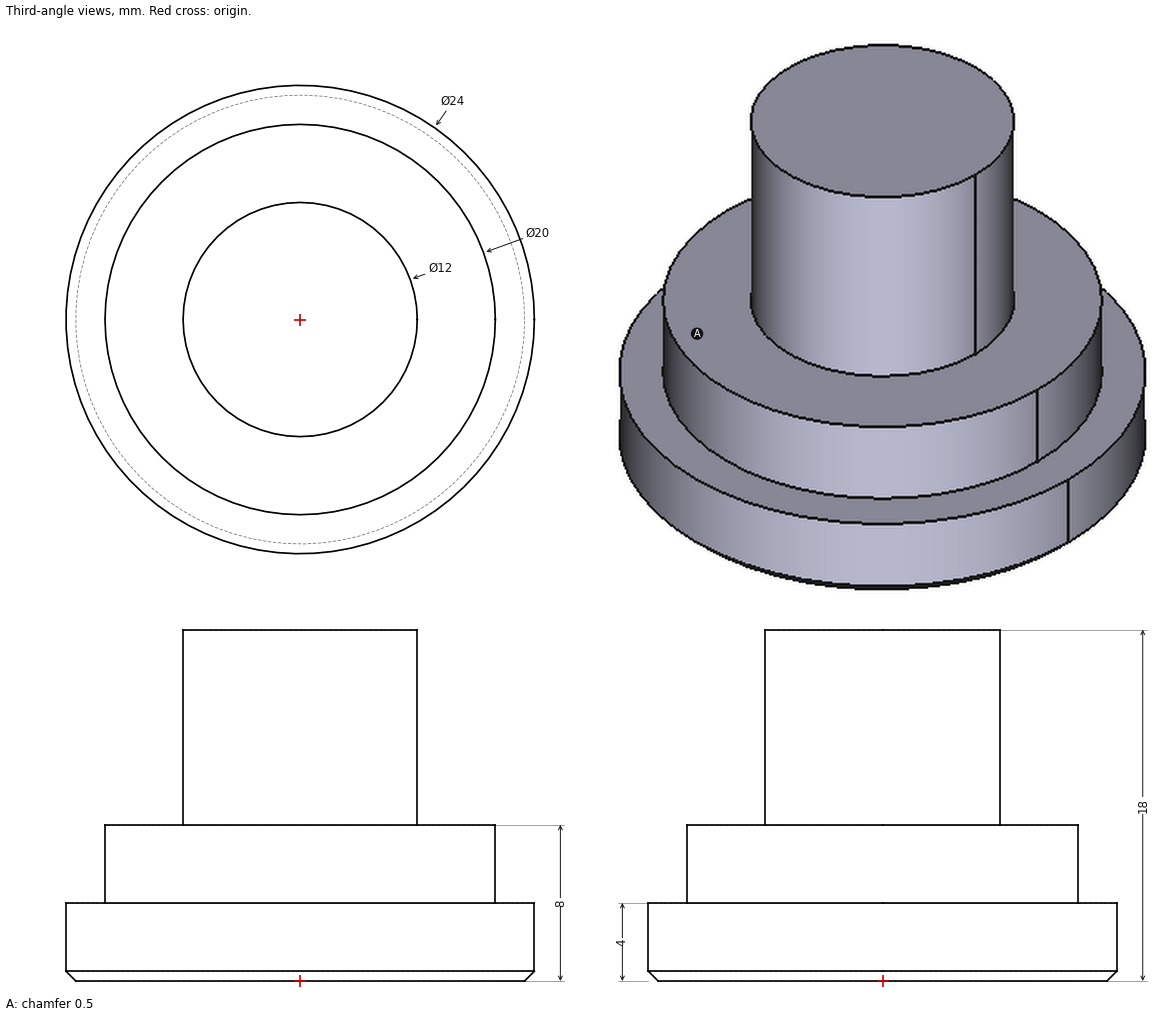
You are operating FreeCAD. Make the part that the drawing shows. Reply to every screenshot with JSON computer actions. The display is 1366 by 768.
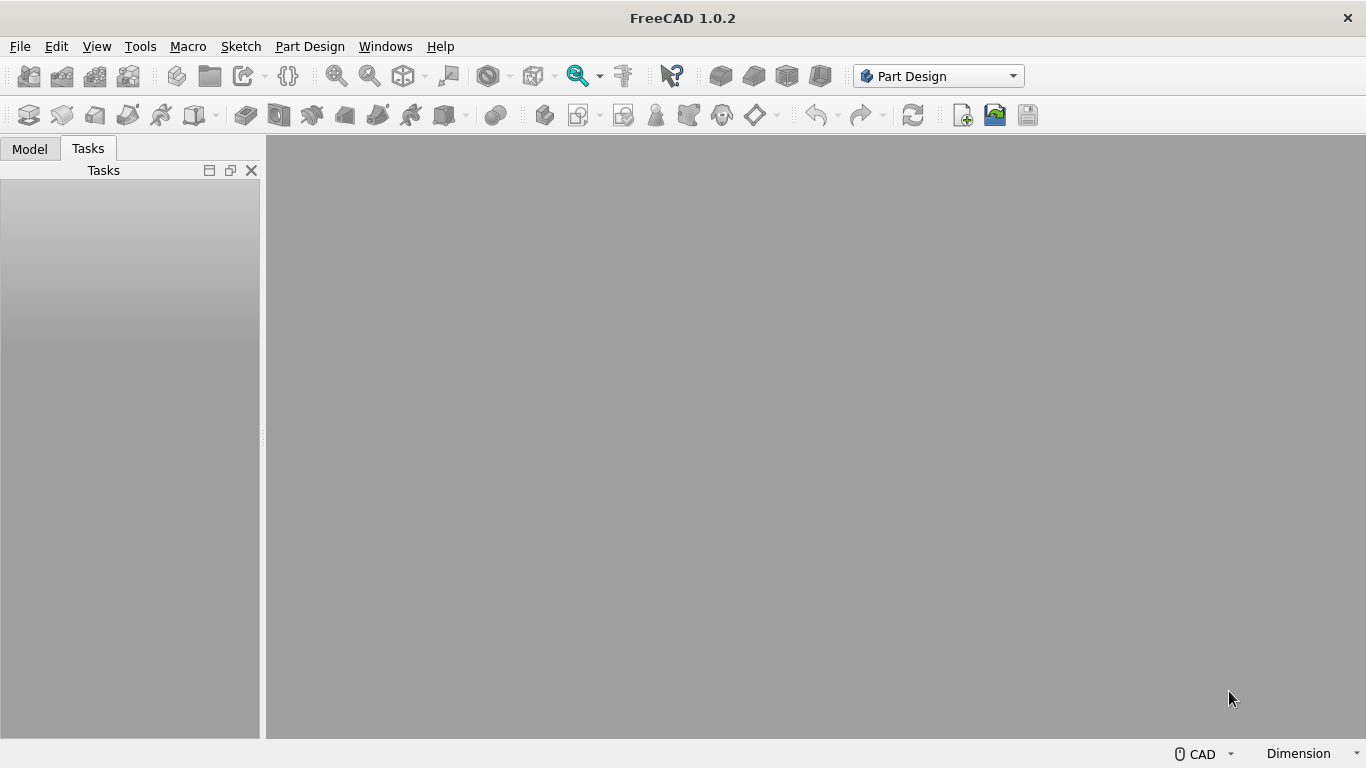
{"action": "left_click", "coordinate": [962, 116]}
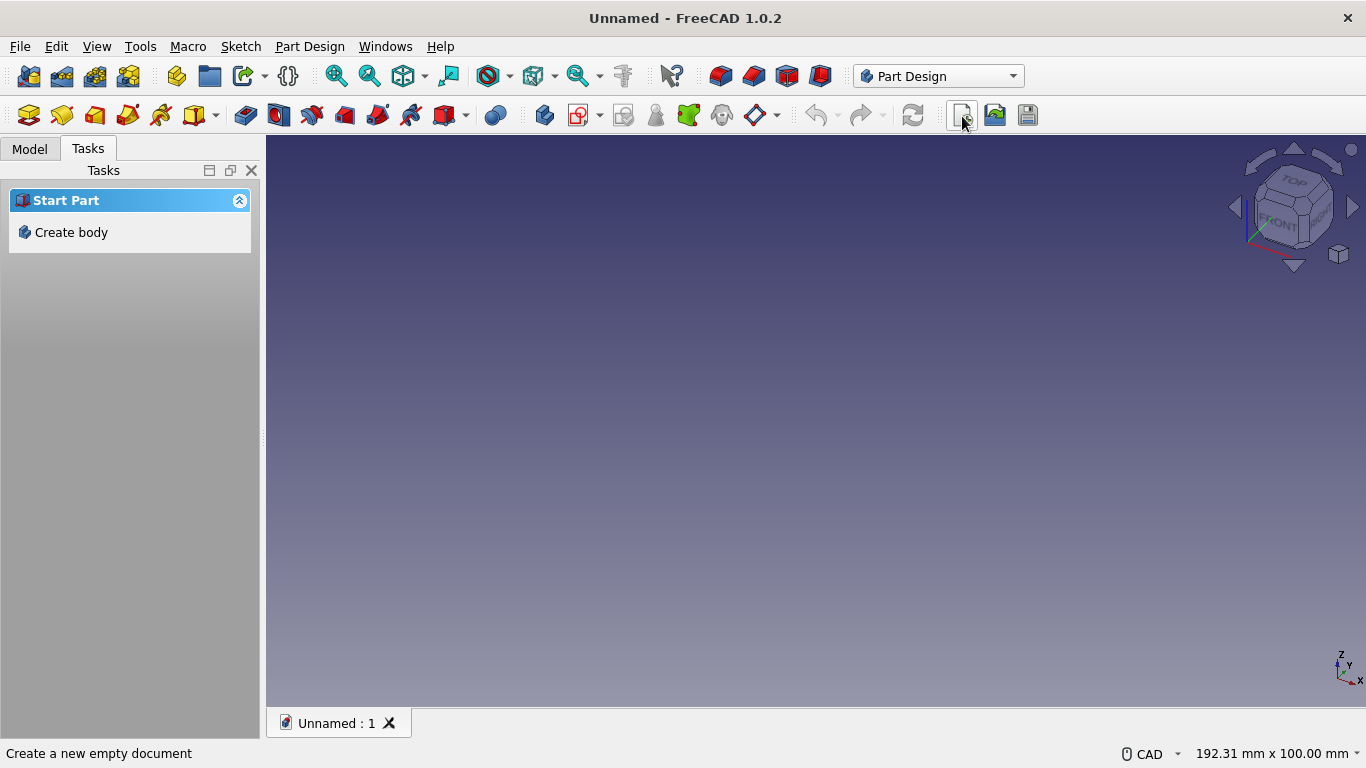
{"action": "left_click", "coordinate": [578, 116]}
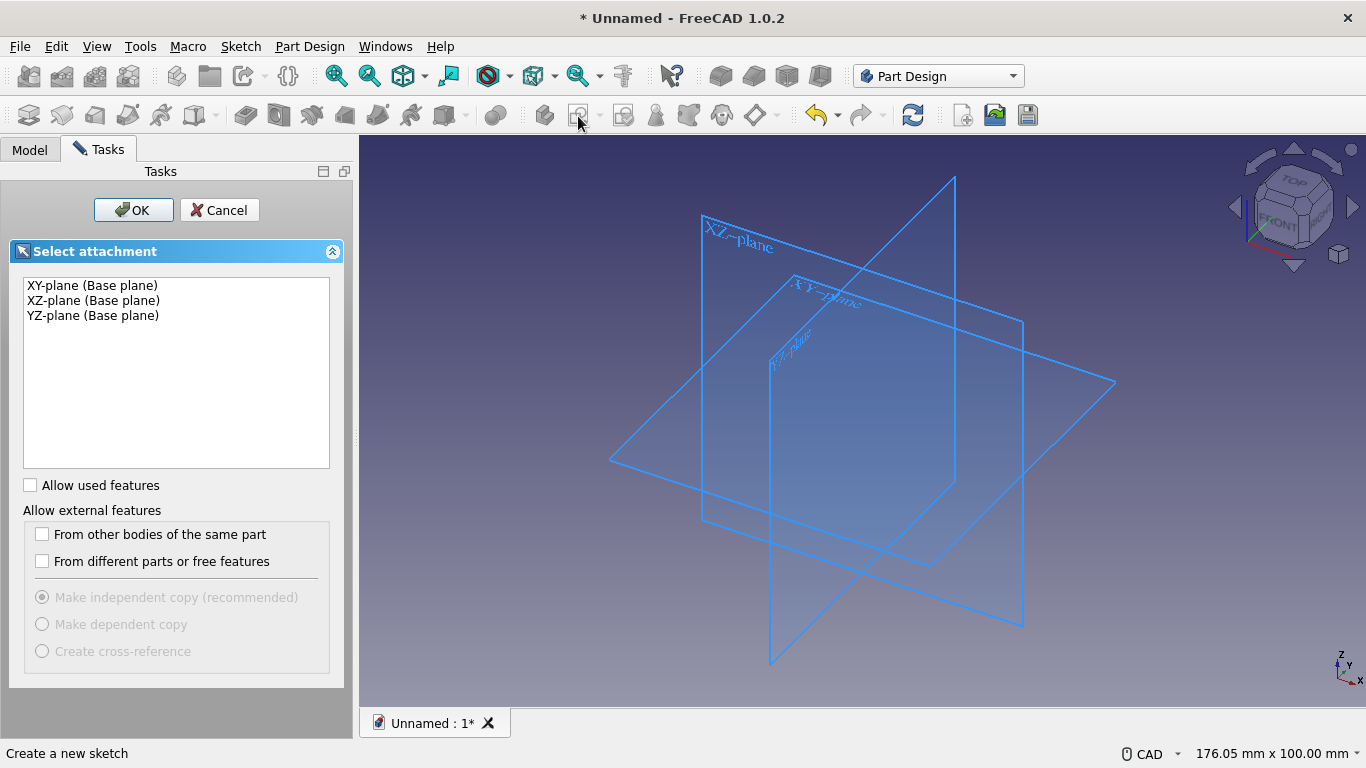
{"action": "left_click", "coordinate": [84, 286]}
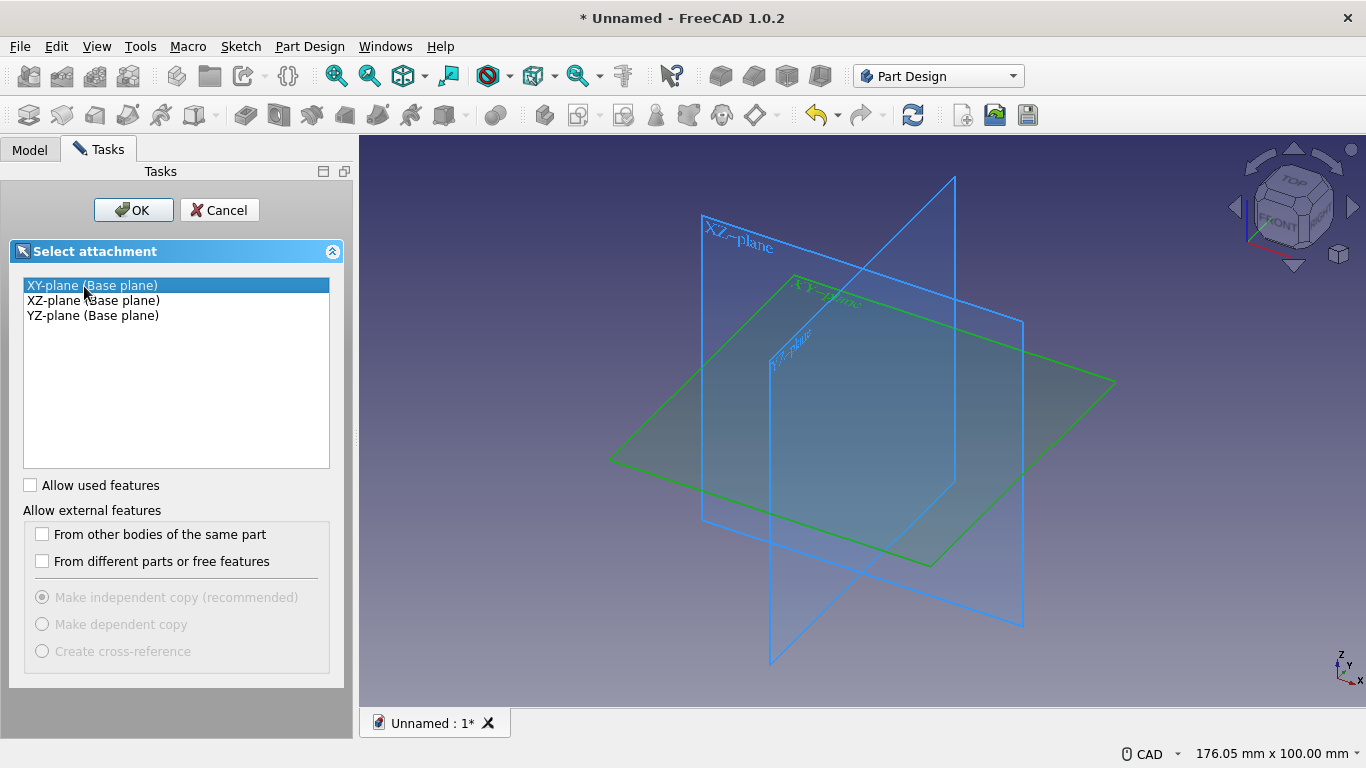
{"action": "left_click", "coordinate": [134, 210]}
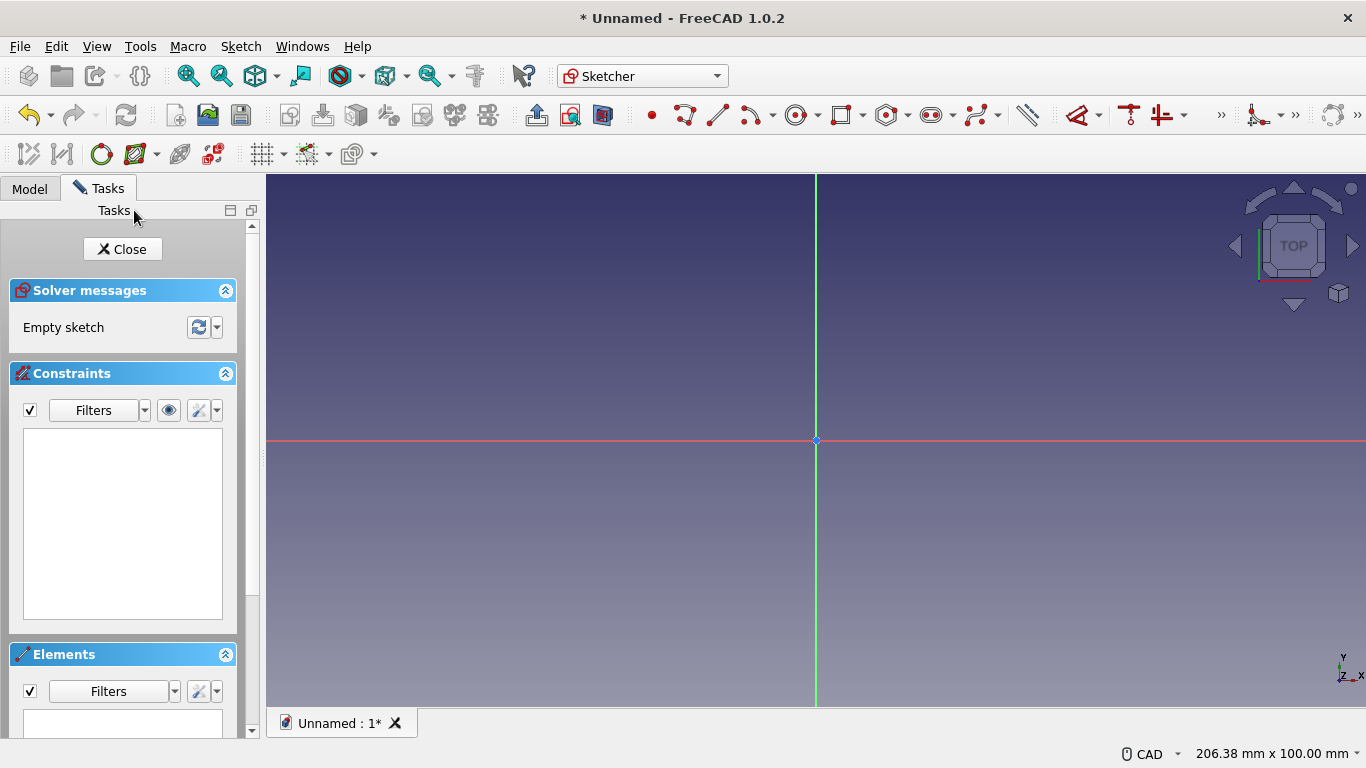
{"action": "scroll", "coordinate": [833, 440], "scroll_direction": "up", "scroll_amount": 8}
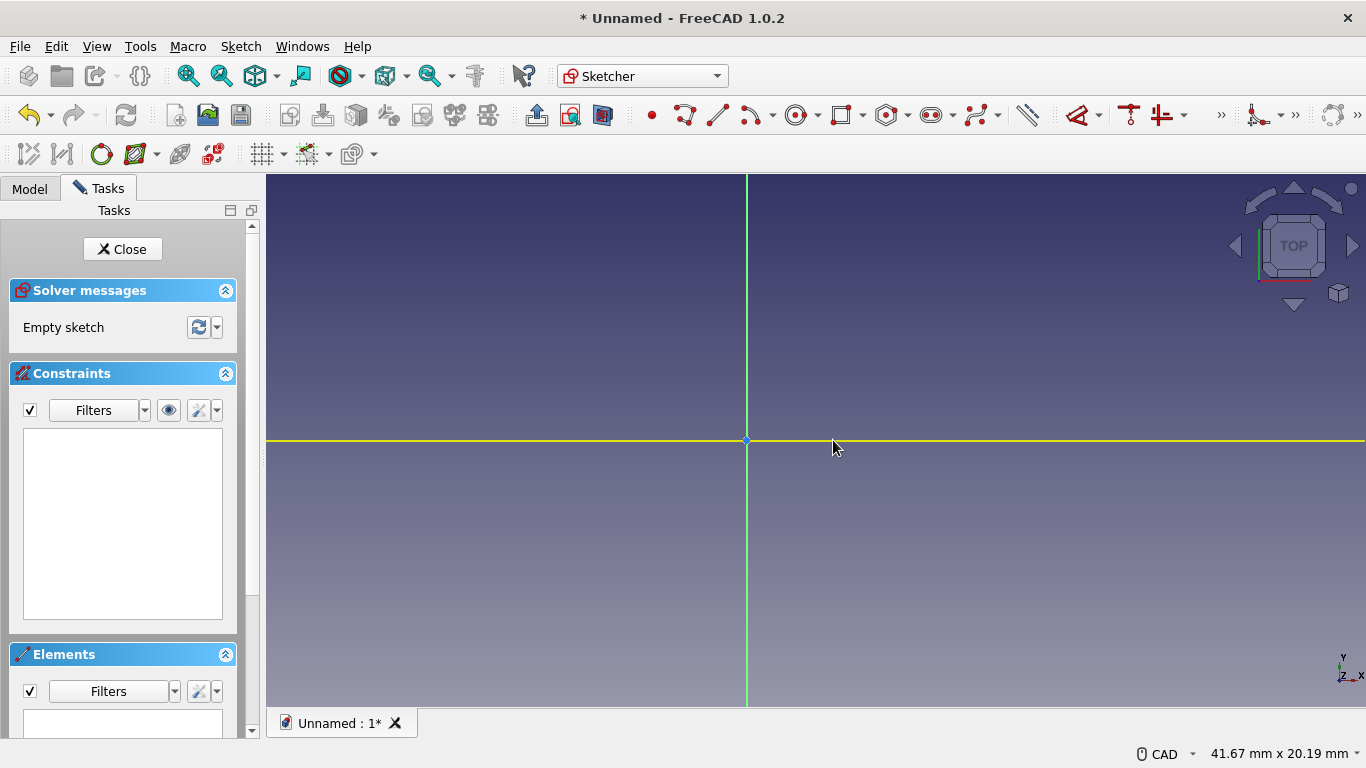
{"action": "left_click", "coordinate": [796, 116]}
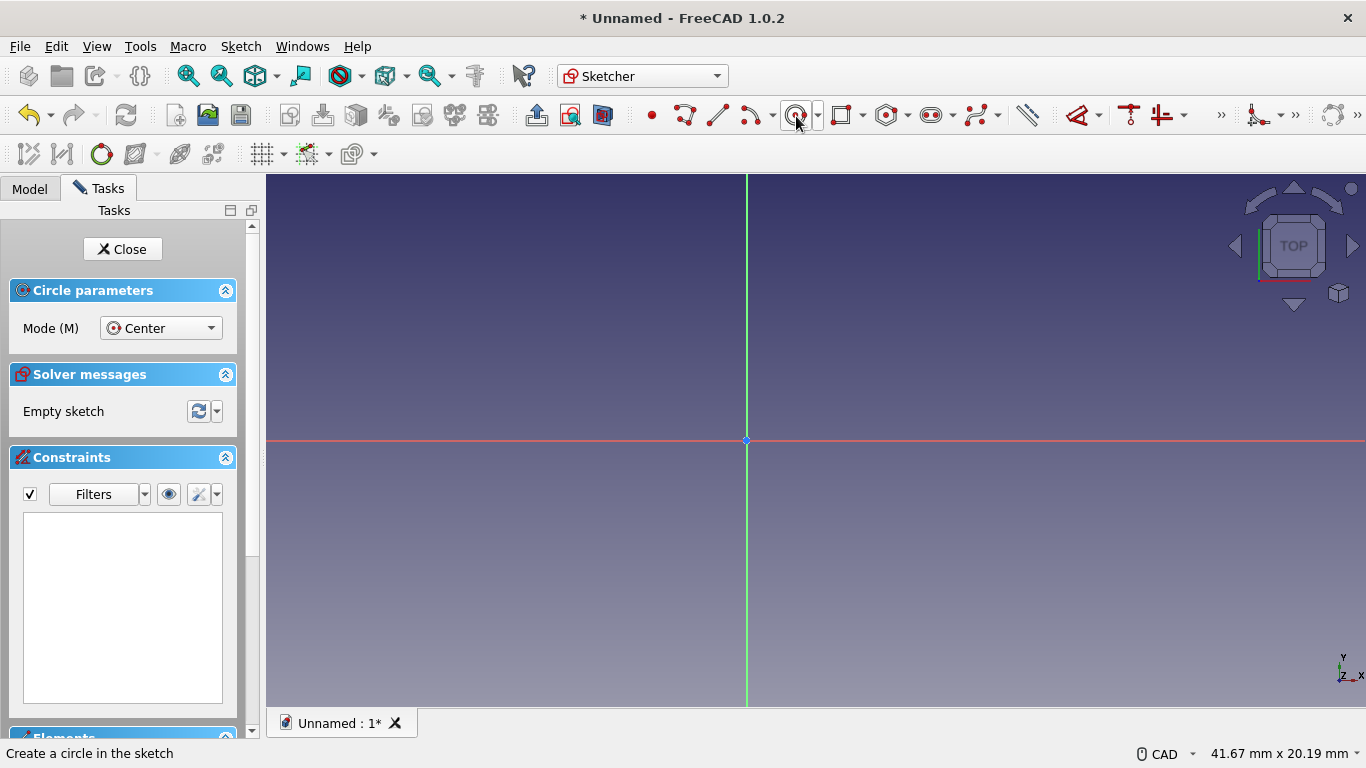
{"action": "left_click", "coordinate": [747, 440]}
{"action": "mouse_move", "coordinate": [859, 328]}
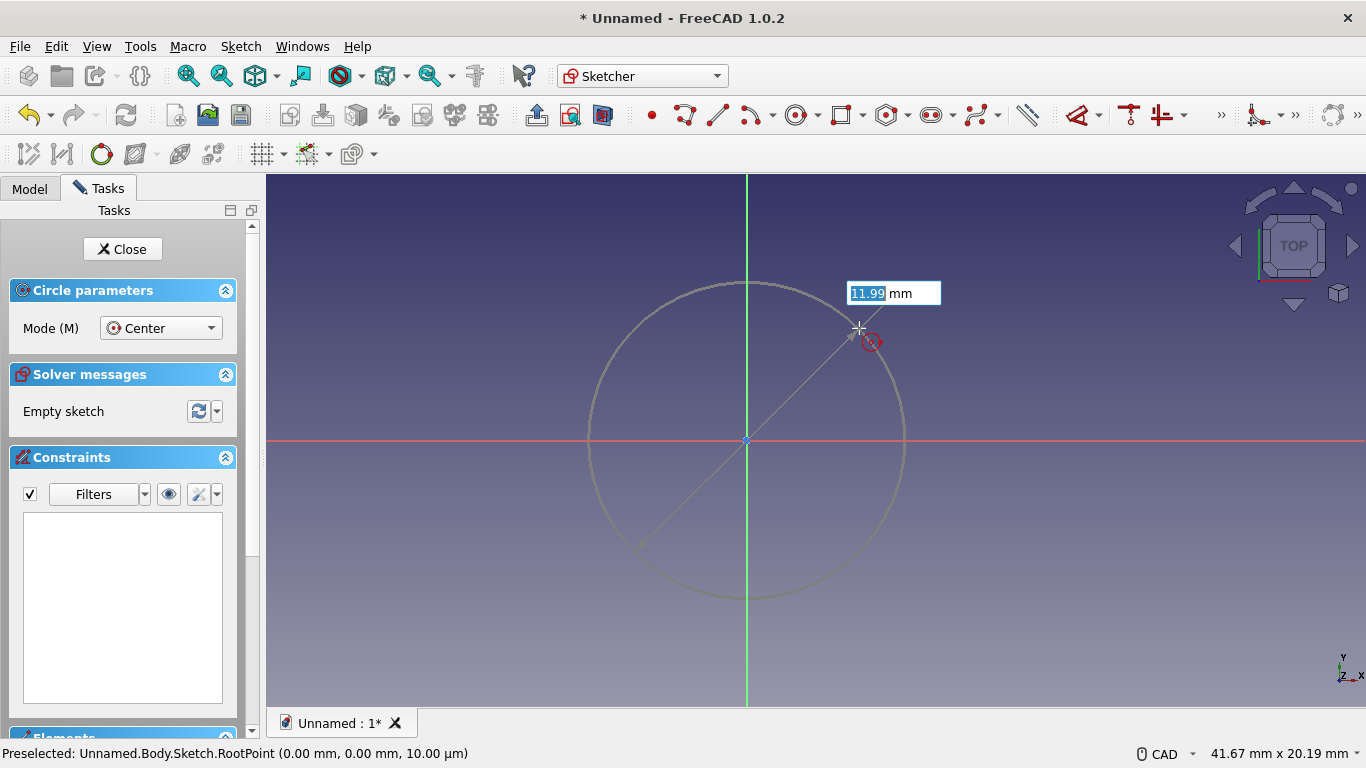
{"action": "type", "text": "12"}
{"action": "key", "text": "Return"}
{"action": "key", "text": "Escape"}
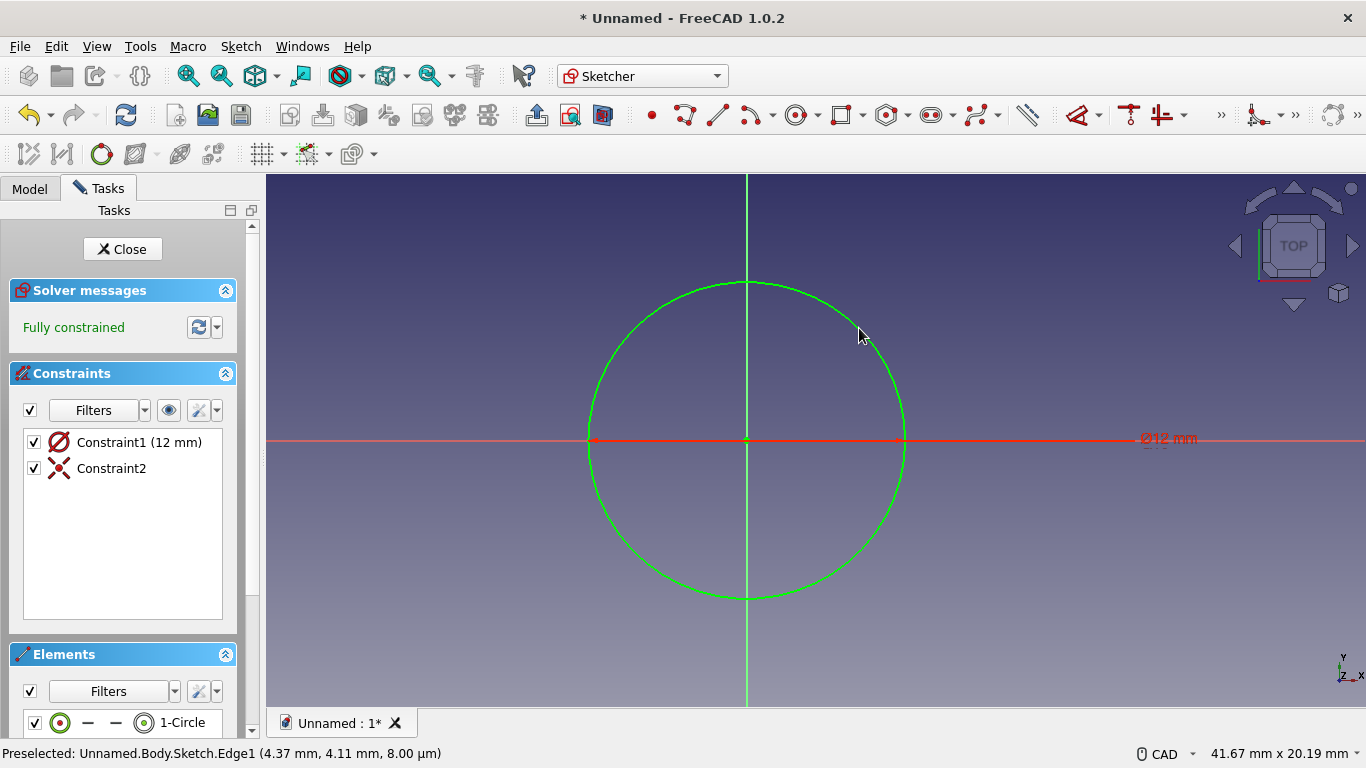
{"action": "left_click", "coordinate": [123, 249]}